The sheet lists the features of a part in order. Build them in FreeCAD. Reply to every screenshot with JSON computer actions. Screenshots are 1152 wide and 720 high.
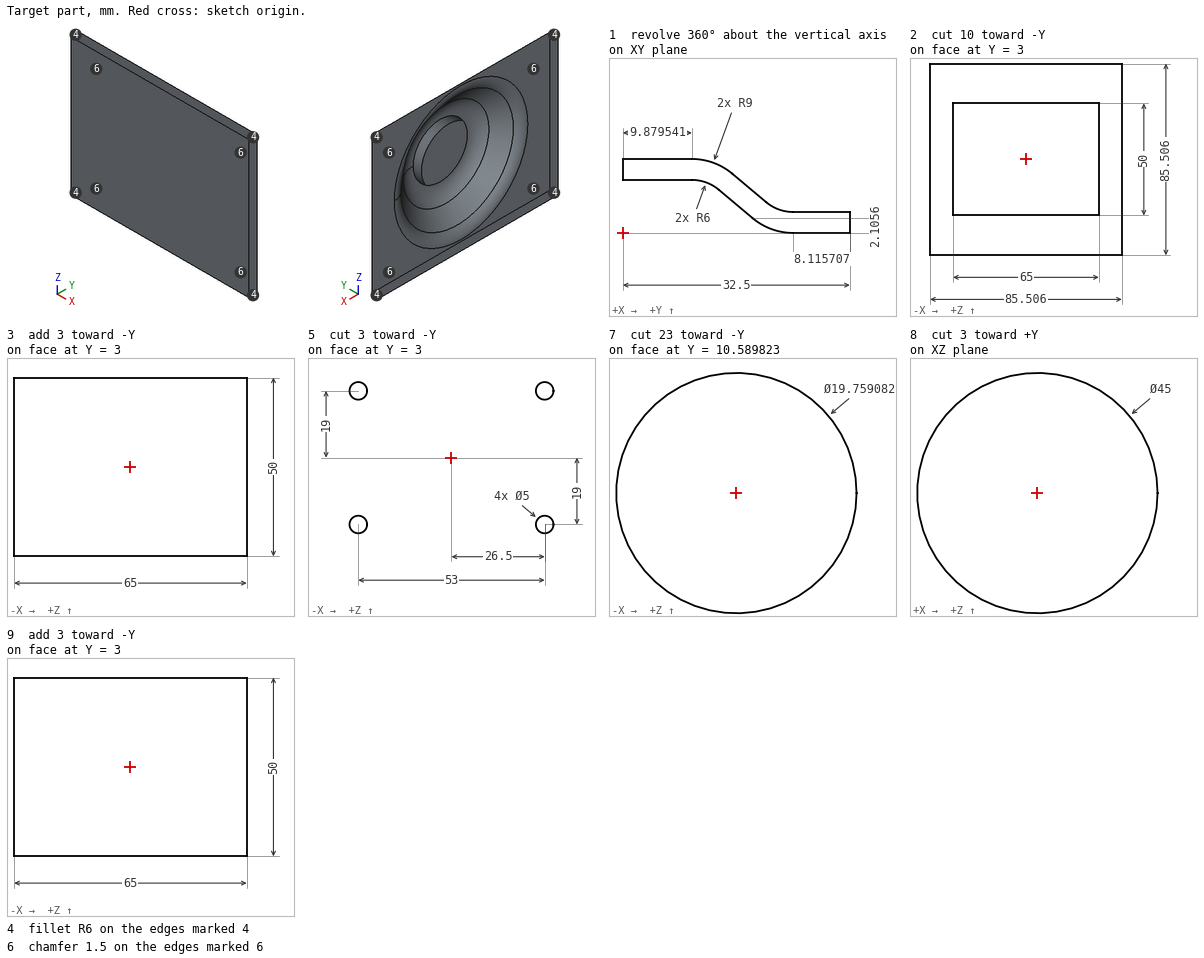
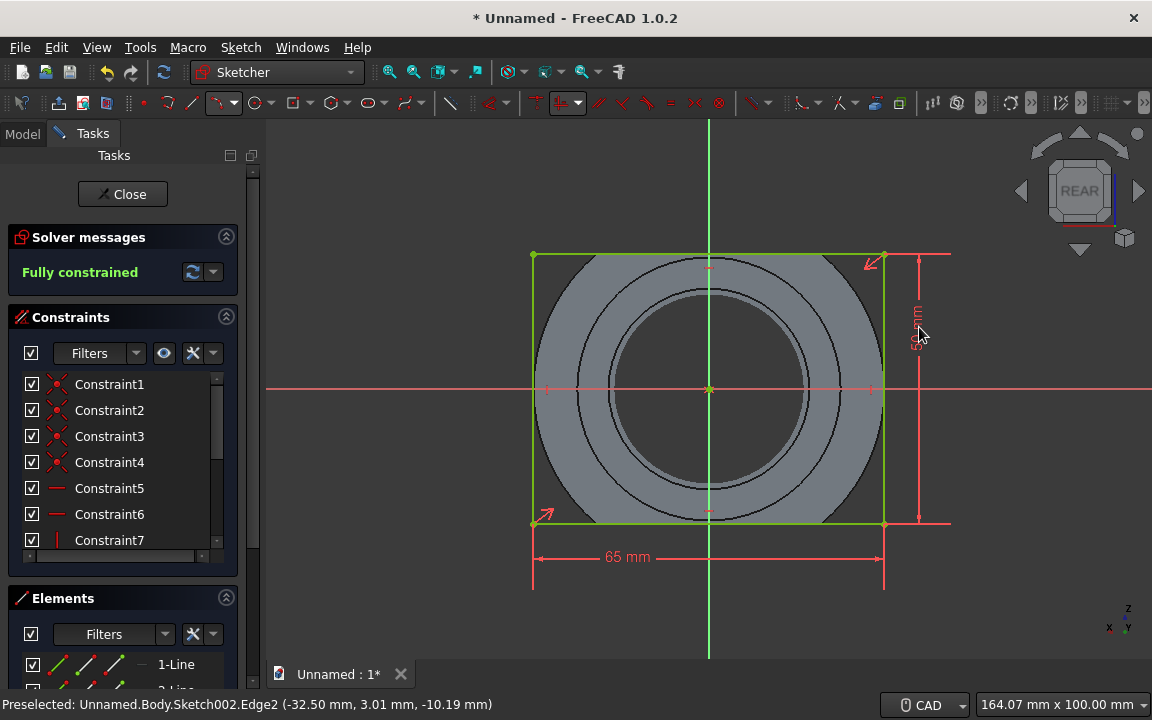
{"action": "left_click", "coordinate": [123, 194]}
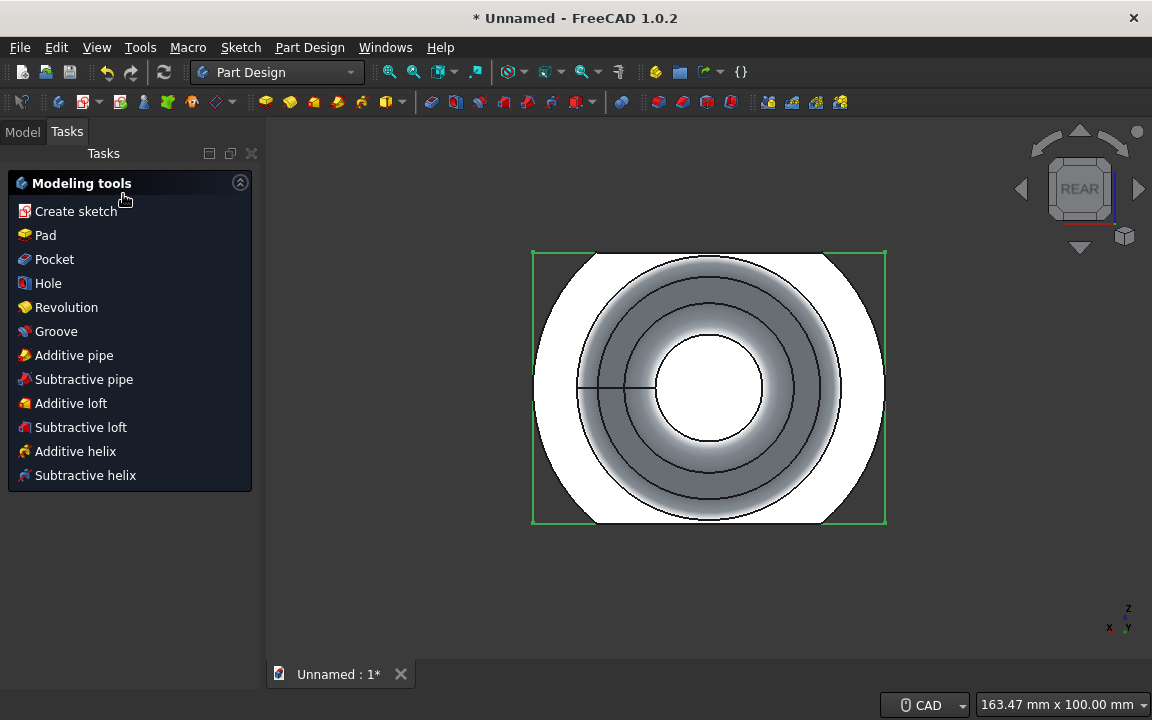
{"action": "left_click", "coordinate": [266, 102]}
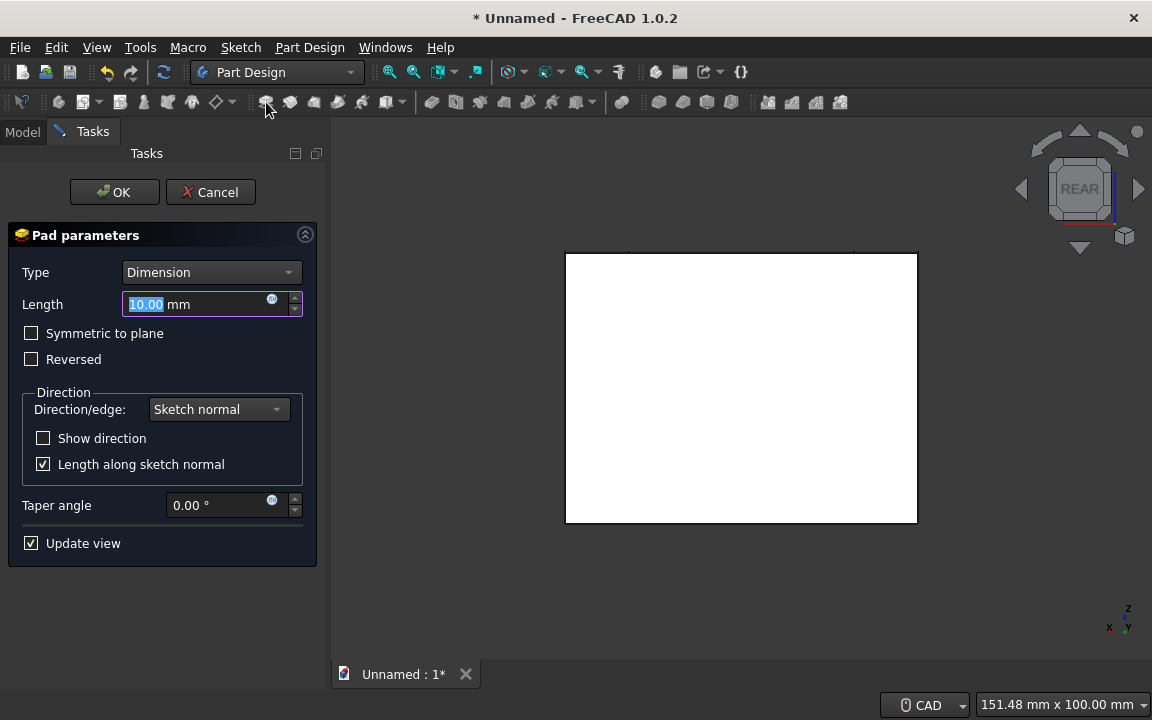
{"action": "type", "text": "3"}
{"action": "key", "text": "Tab"}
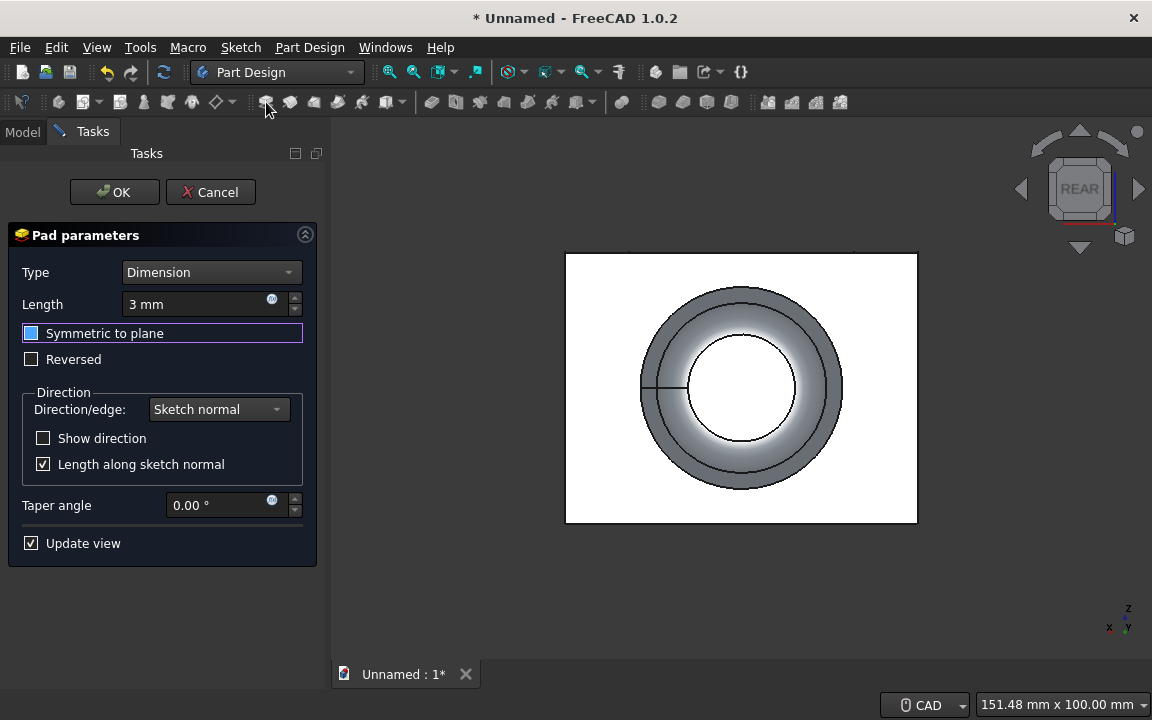
{"action": "left_click", "coordinate": [30, 359]}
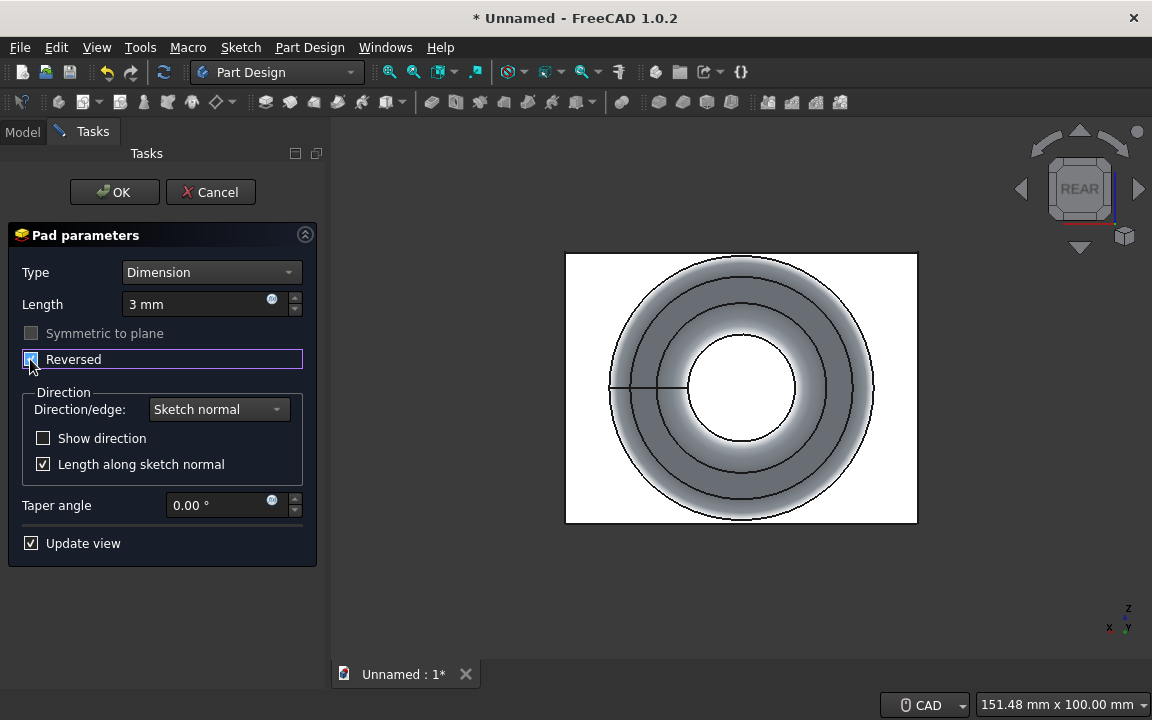
{"action": "left_click", "coordinate": [115, 192]}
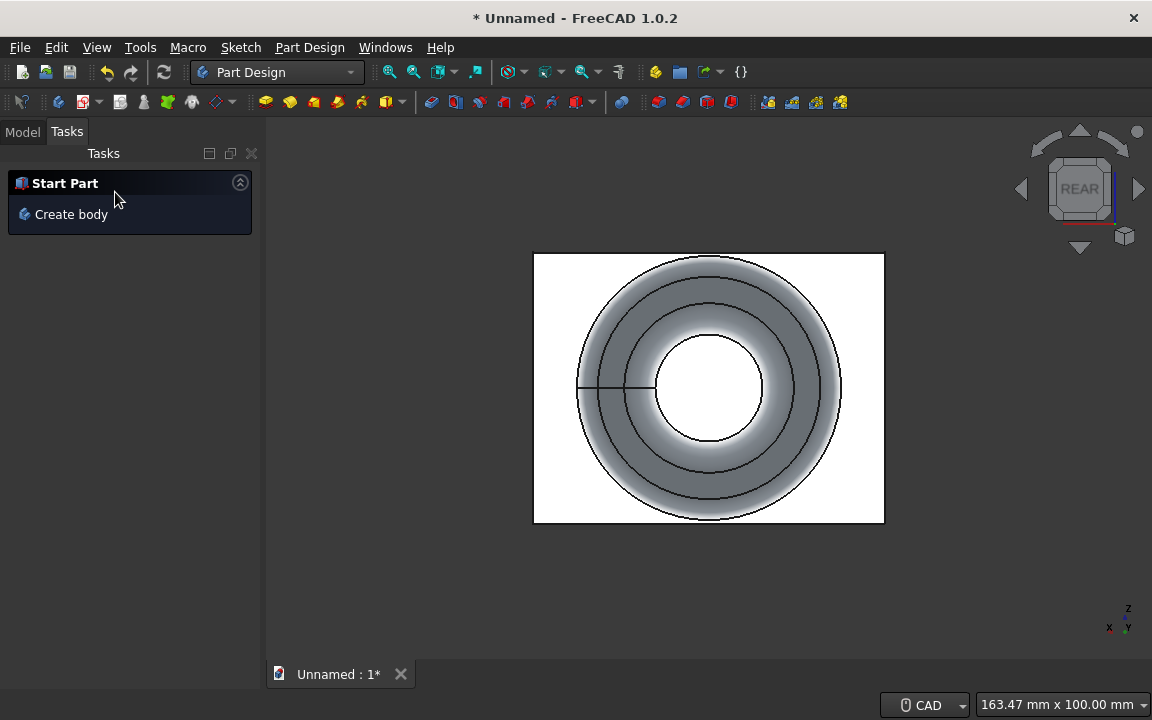
{"action": "scroll", "coordinate": [533, 523], "scroll_direction": "up", "scroll_amount": 5}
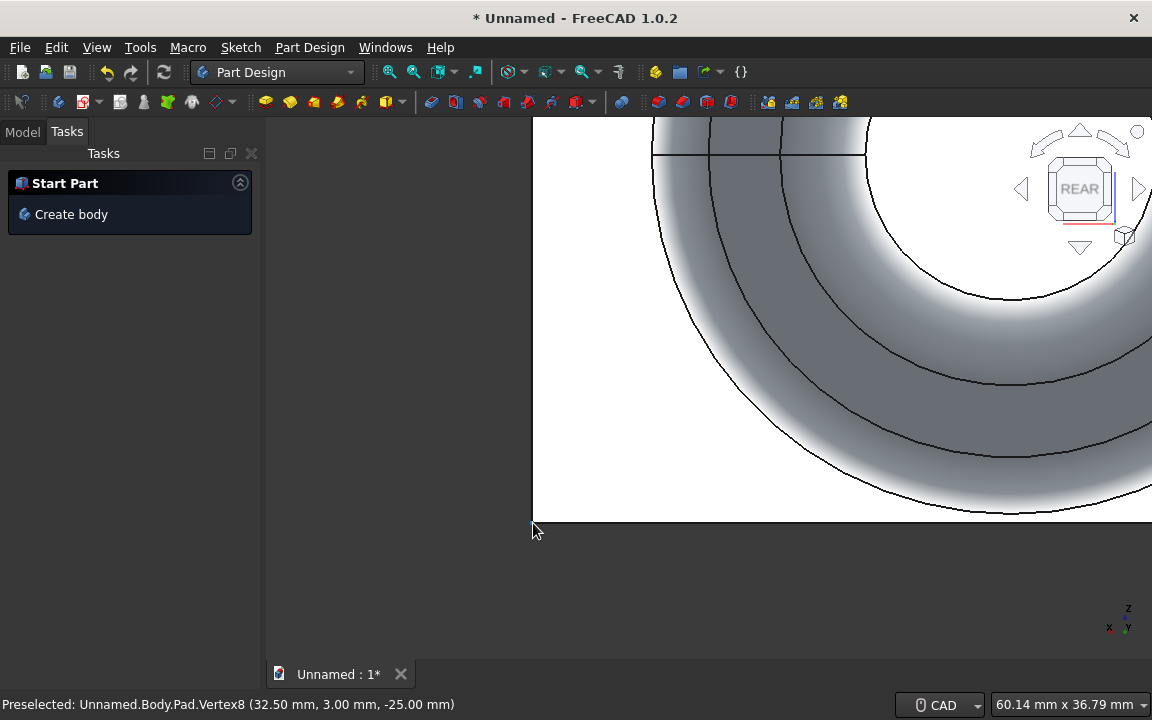
{"action": "left_click", "coordinate": [390, 72]}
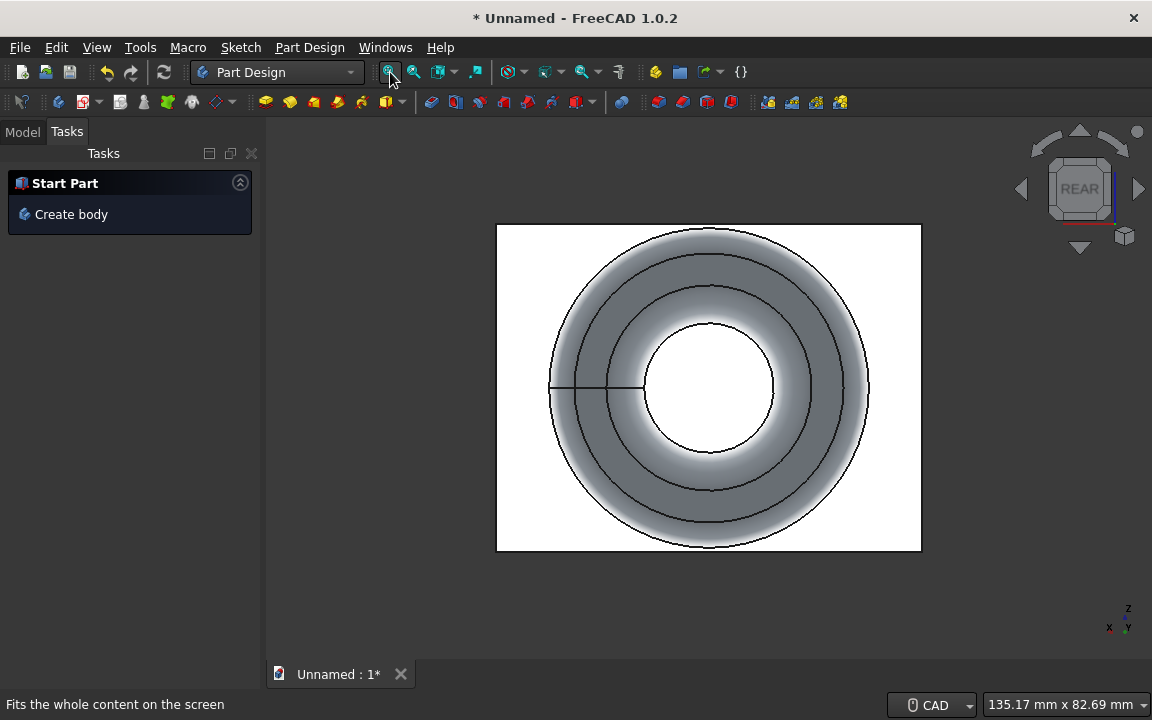
{"action": "key", "text": "0"}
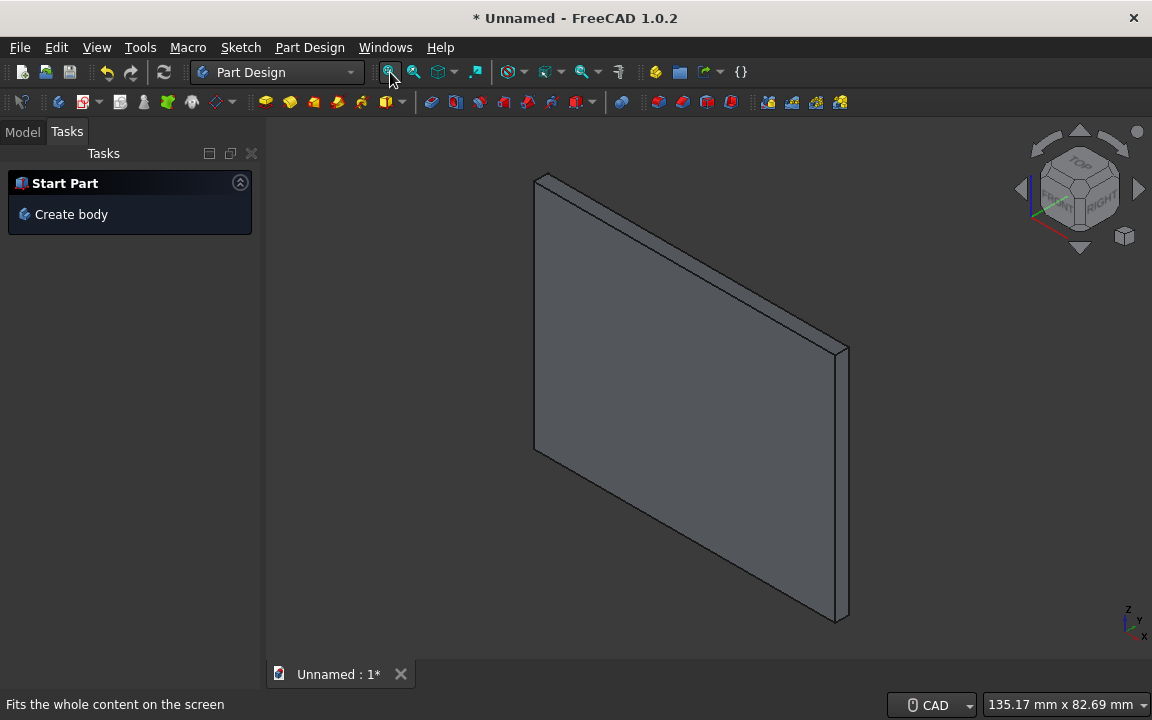
{"action": "left_click", "coordinate": [842, 350]}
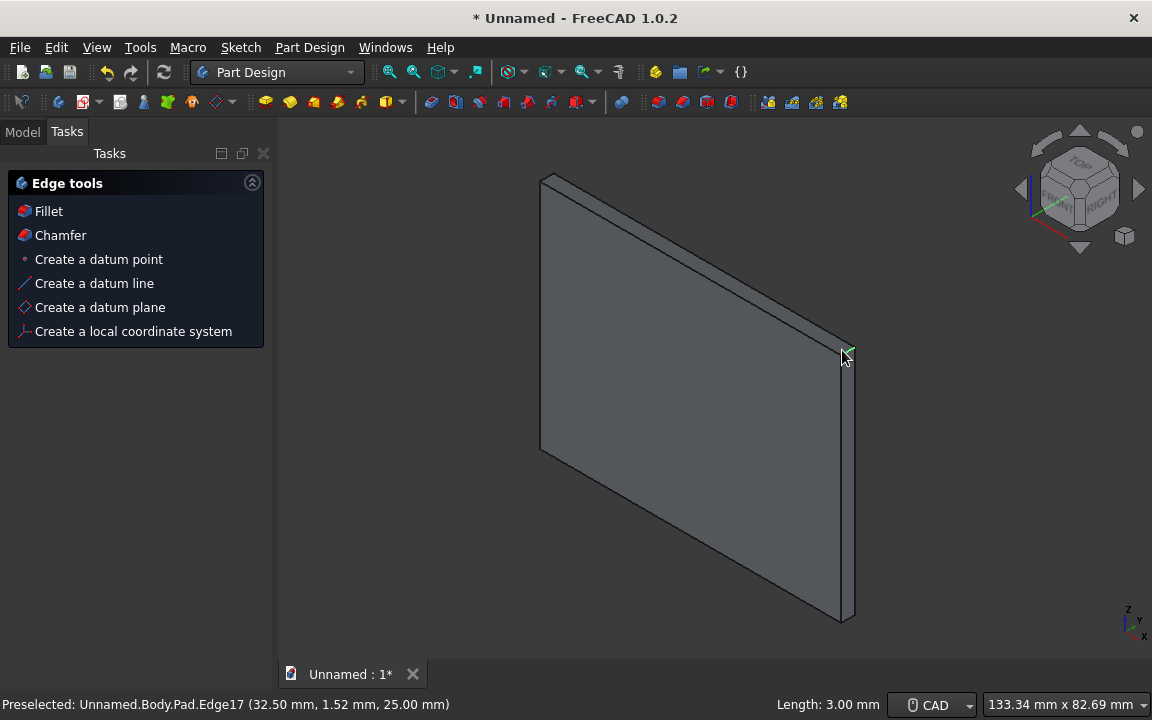
{"action": "scroll", "coordinate": [848, 618], "scroll_direction": "up", "scroll_amount": 4}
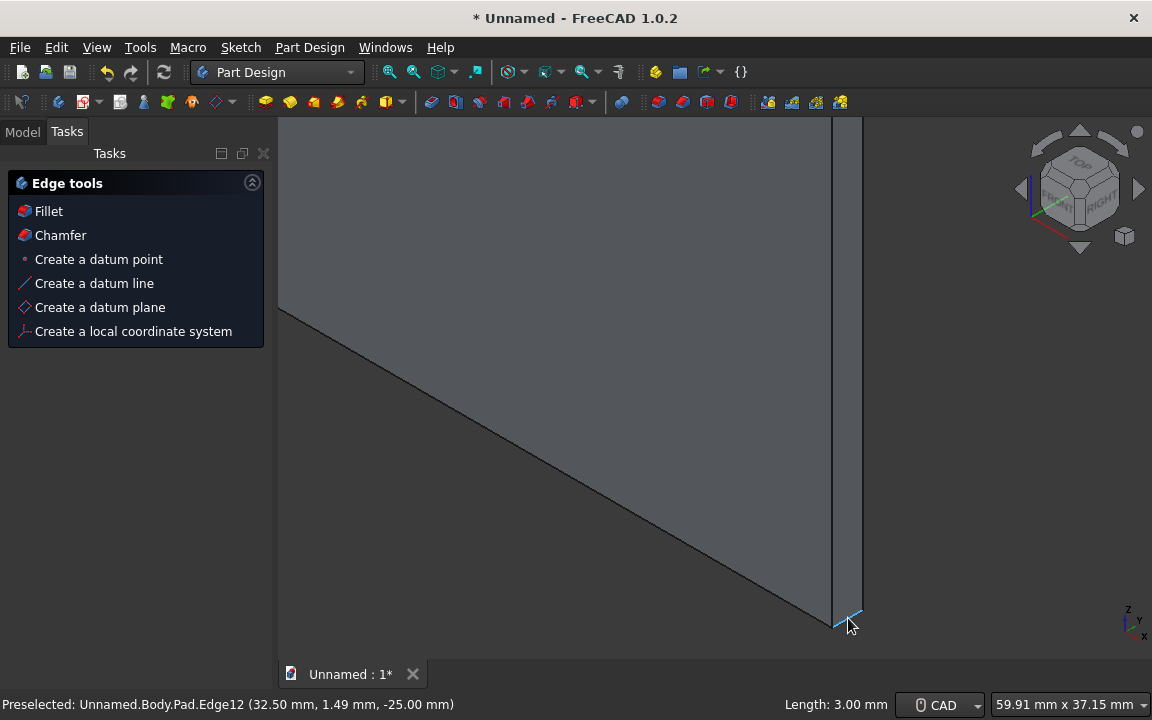
{"action": "left_click", "coordinate": [390, 72]}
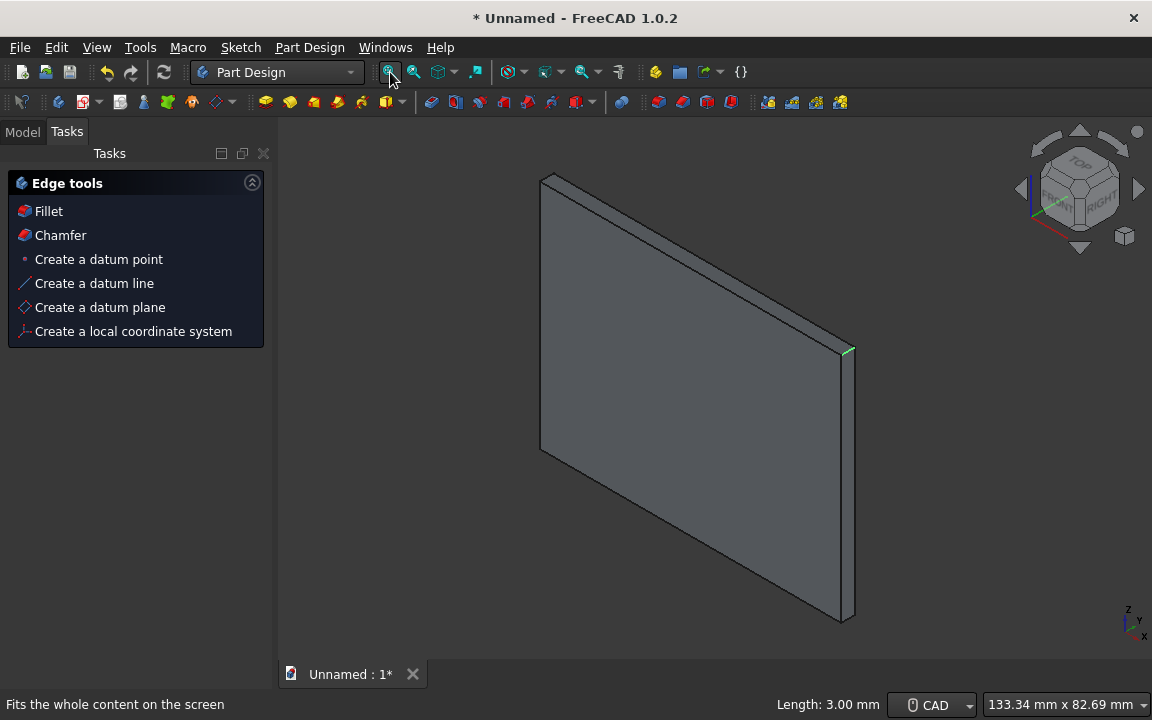
{"action": "key", "text": "2"}